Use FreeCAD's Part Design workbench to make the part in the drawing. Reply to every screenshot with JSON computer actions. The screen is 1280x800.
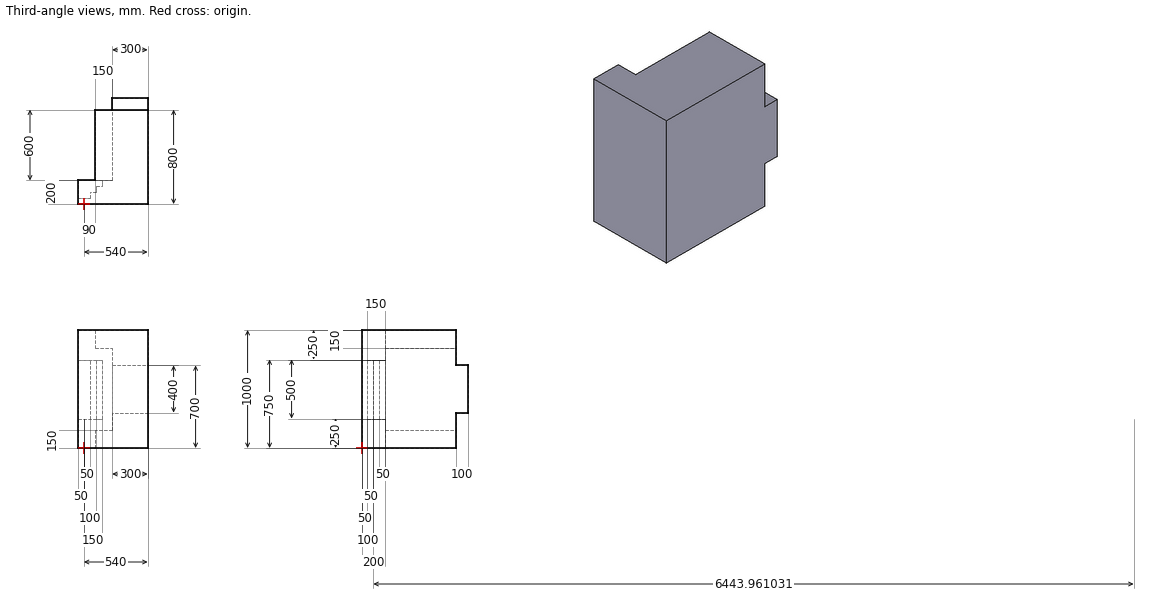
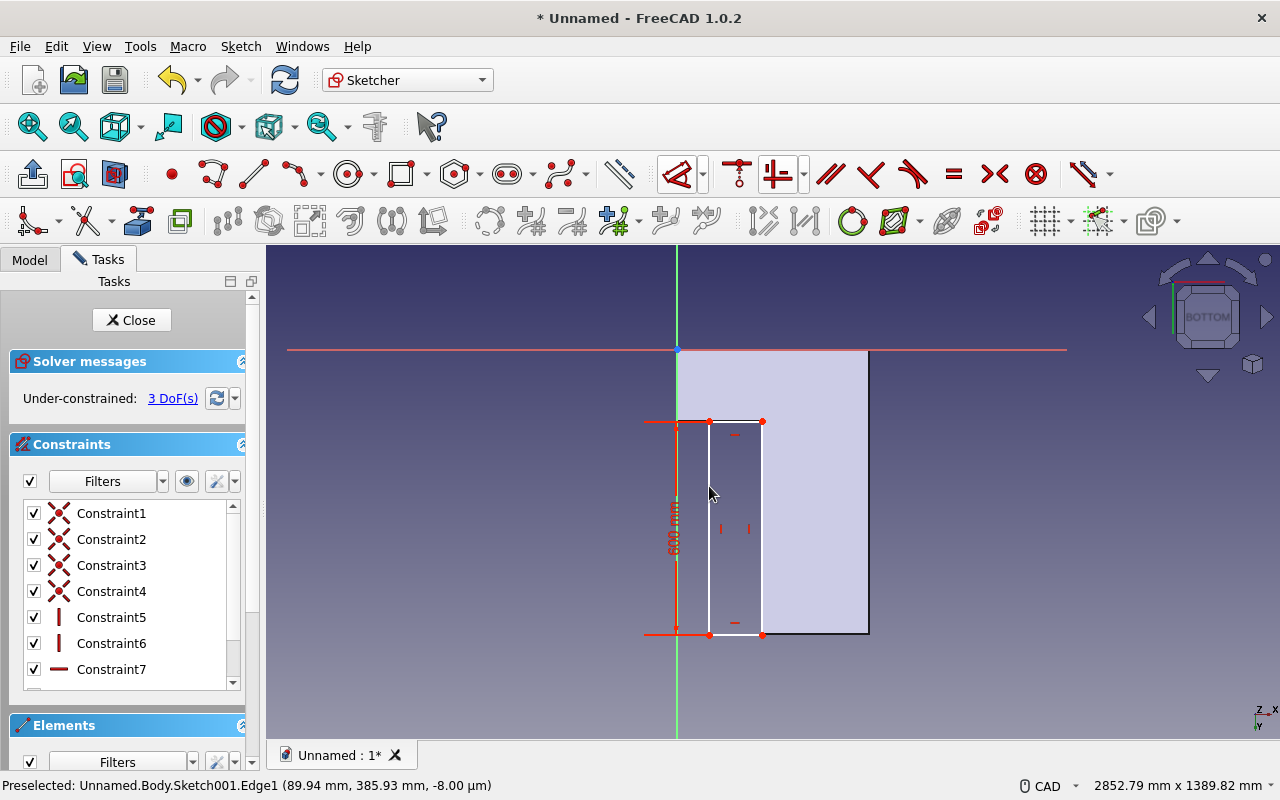
{"action": "left_click", "coordinate": [725, 635]}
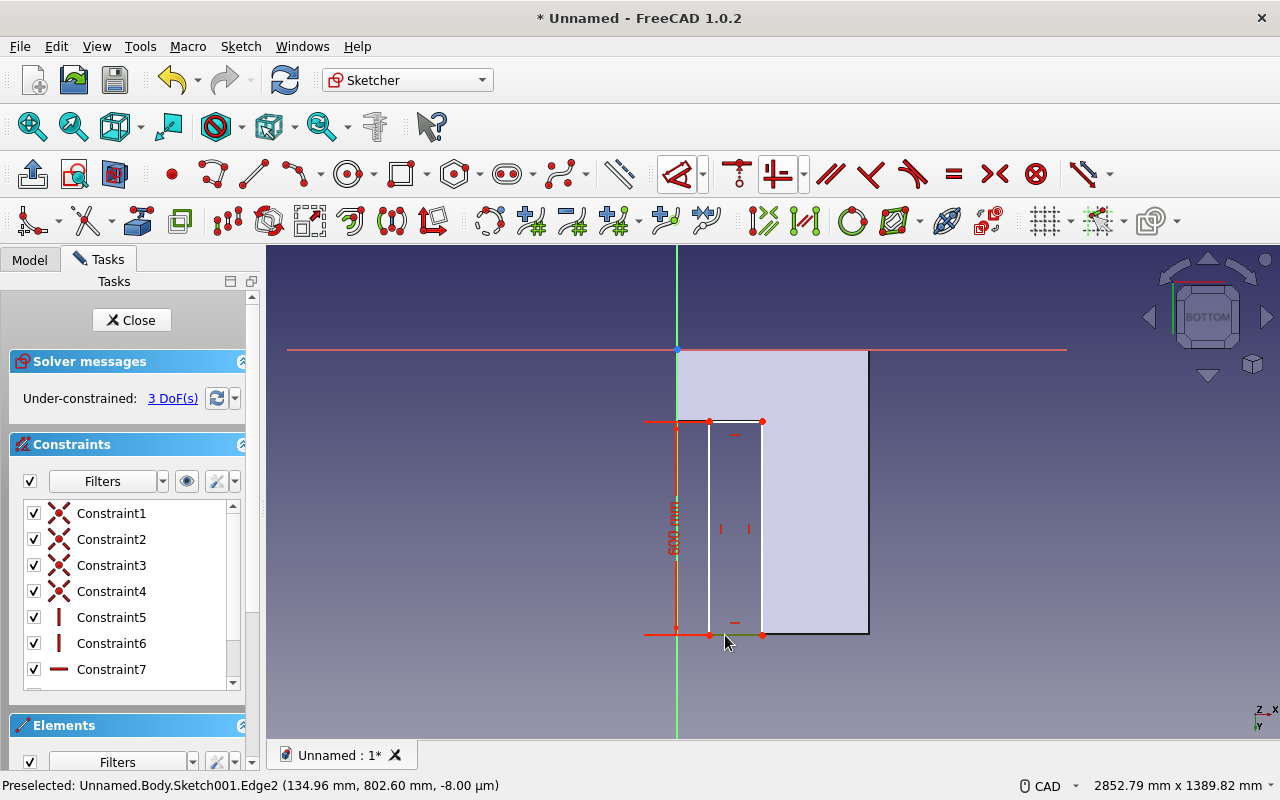
{"action": "left_click", "coordinate": [702, 174]}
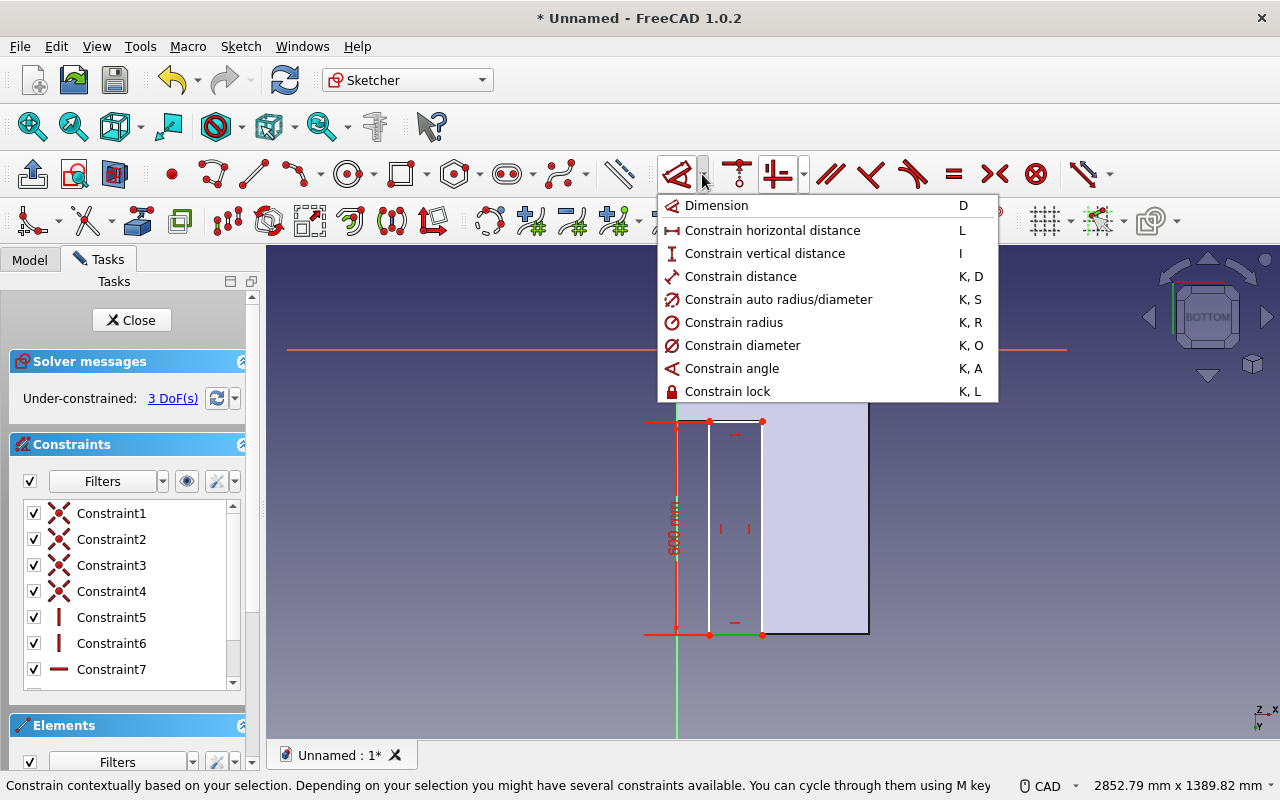
{"action": "left_click", "coordinate": [828, 230]}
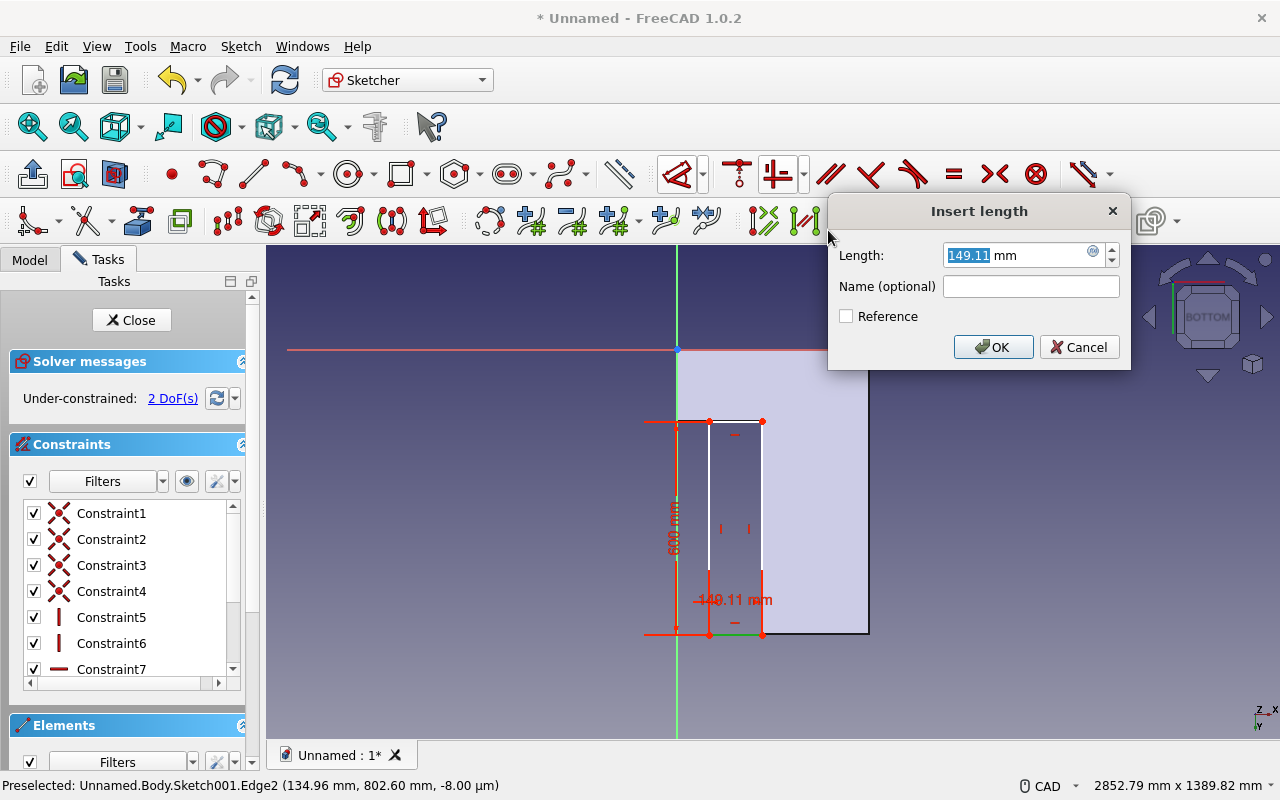
{"action": "type", "text": "150"}
{"action": "key", "text": "Return"}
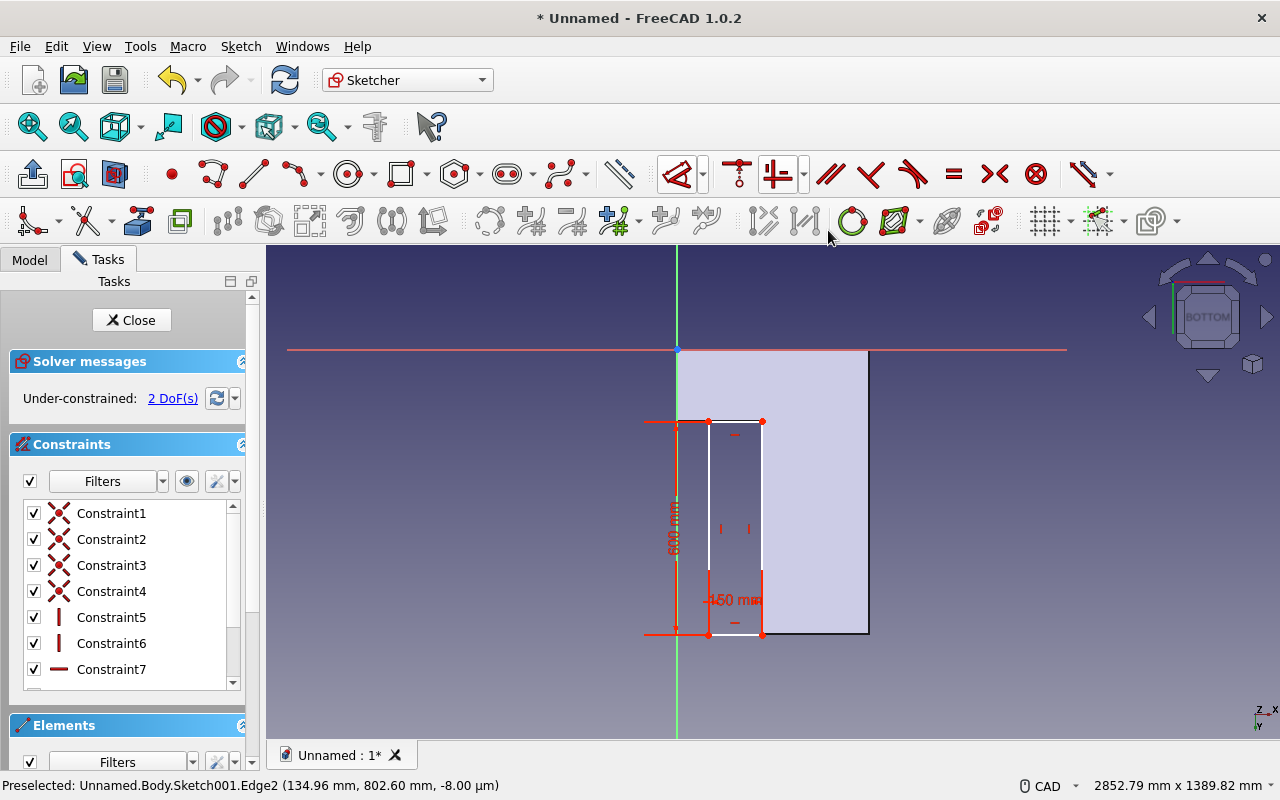
{"action": "scroll", "coordinate": [709, 422], "scroll_direction": "up", "scroll_amount": 2}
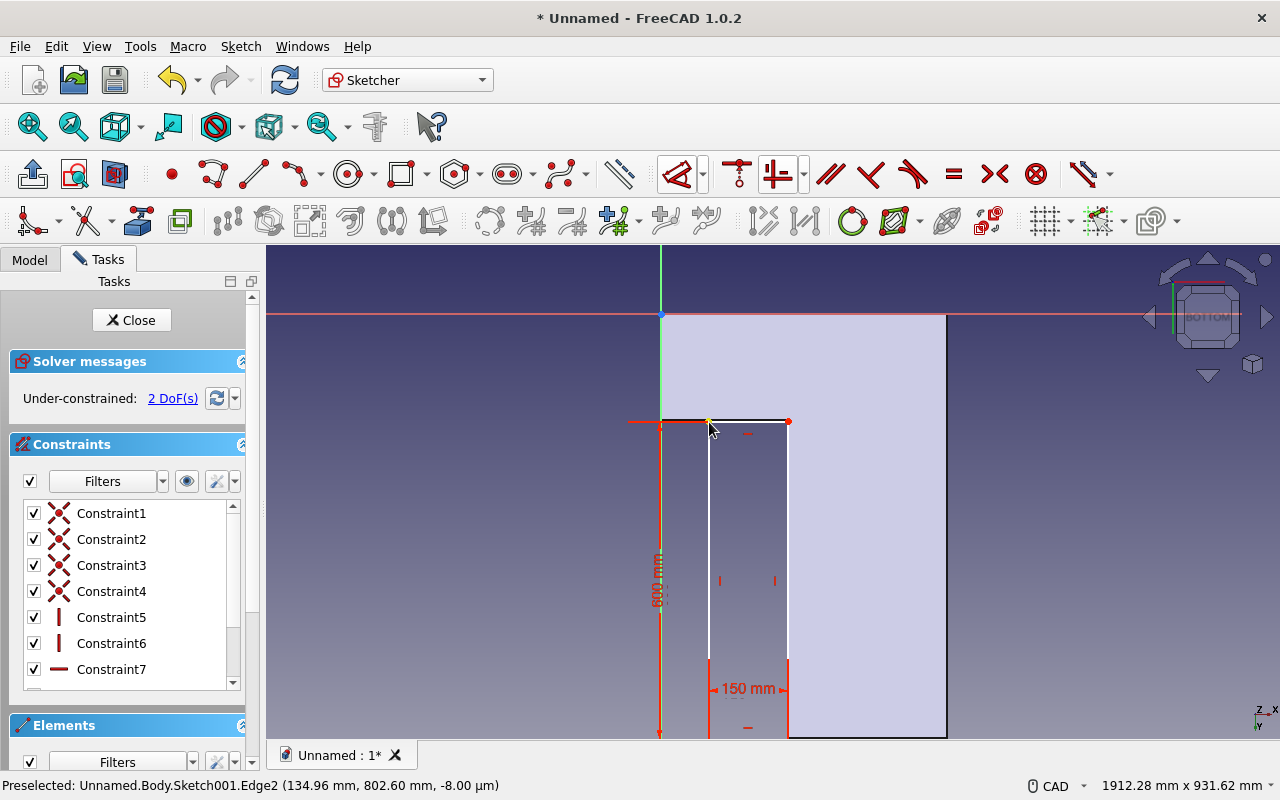
{"action": "left_click", "coordinate": [709, 422]}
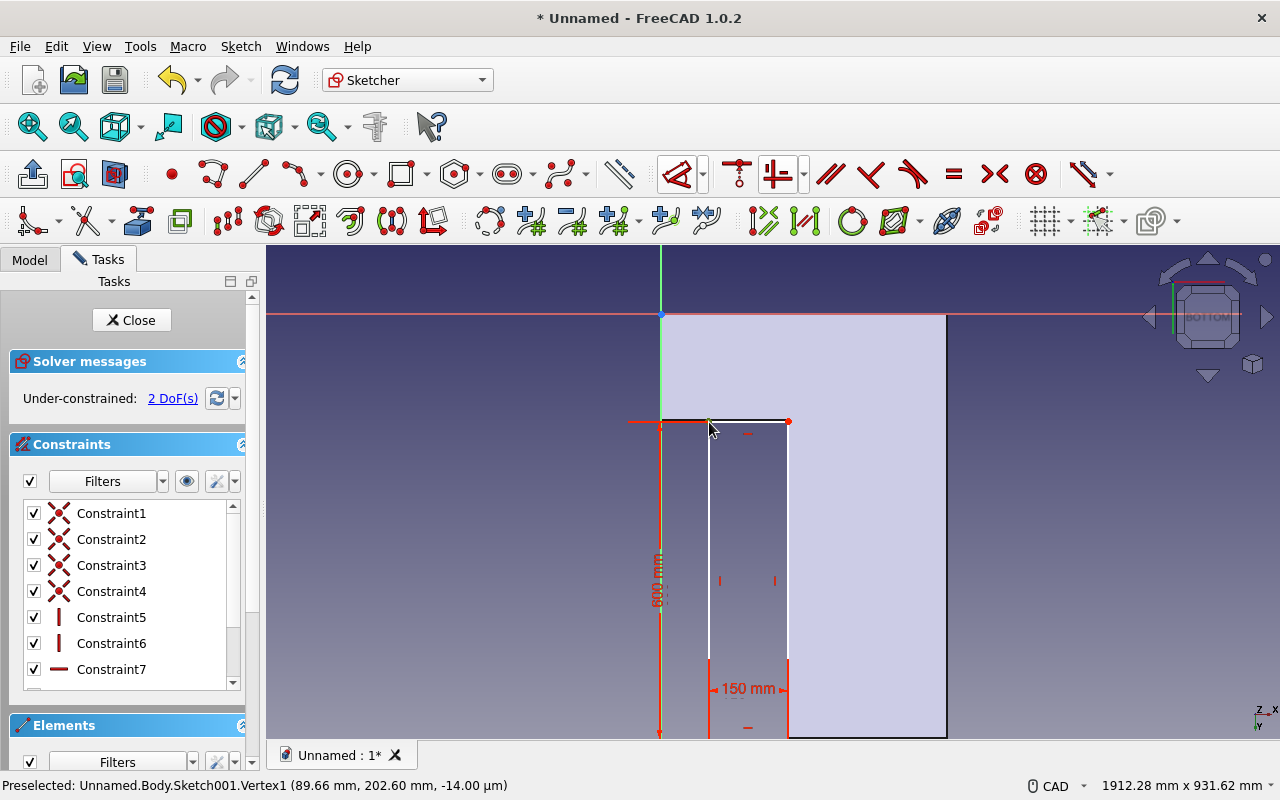
{"action": "key", "text": "l"}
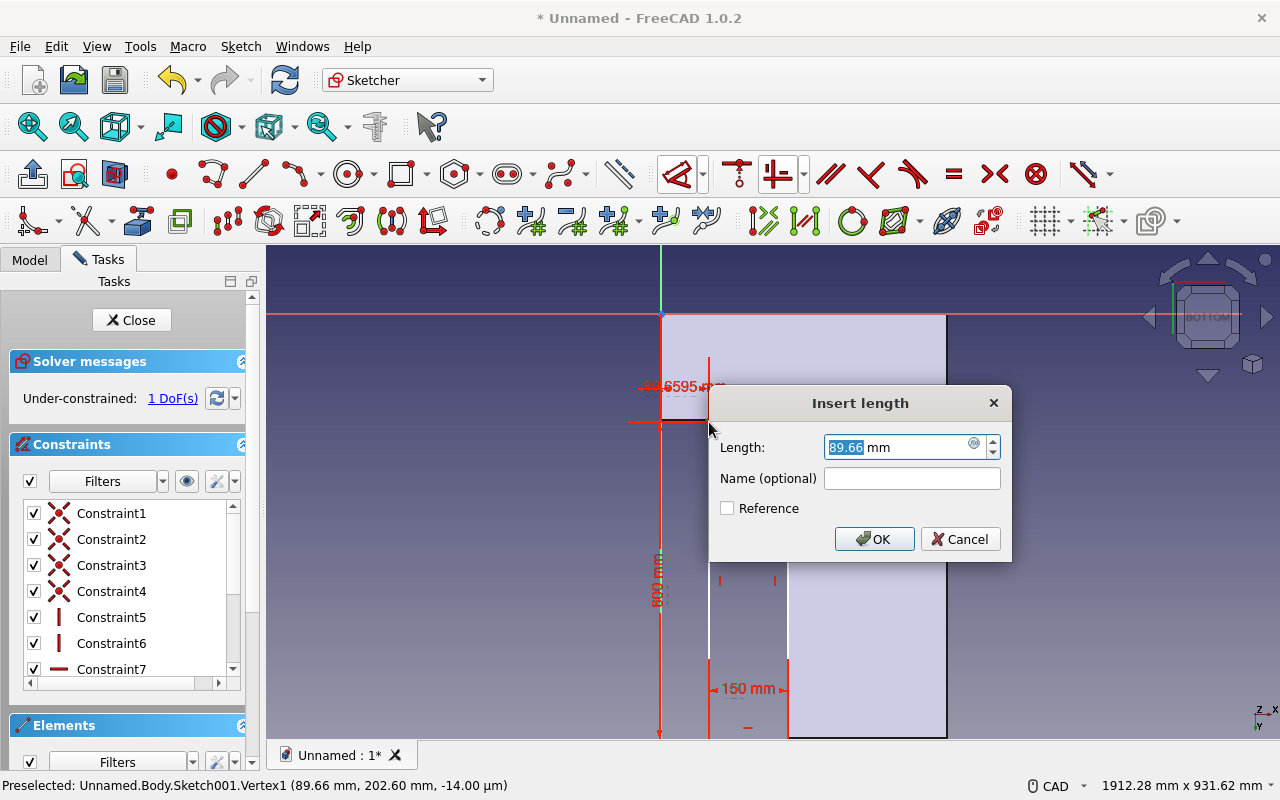
{"action": "type", "text": "90"}
{"action": "key", "text": "Return"}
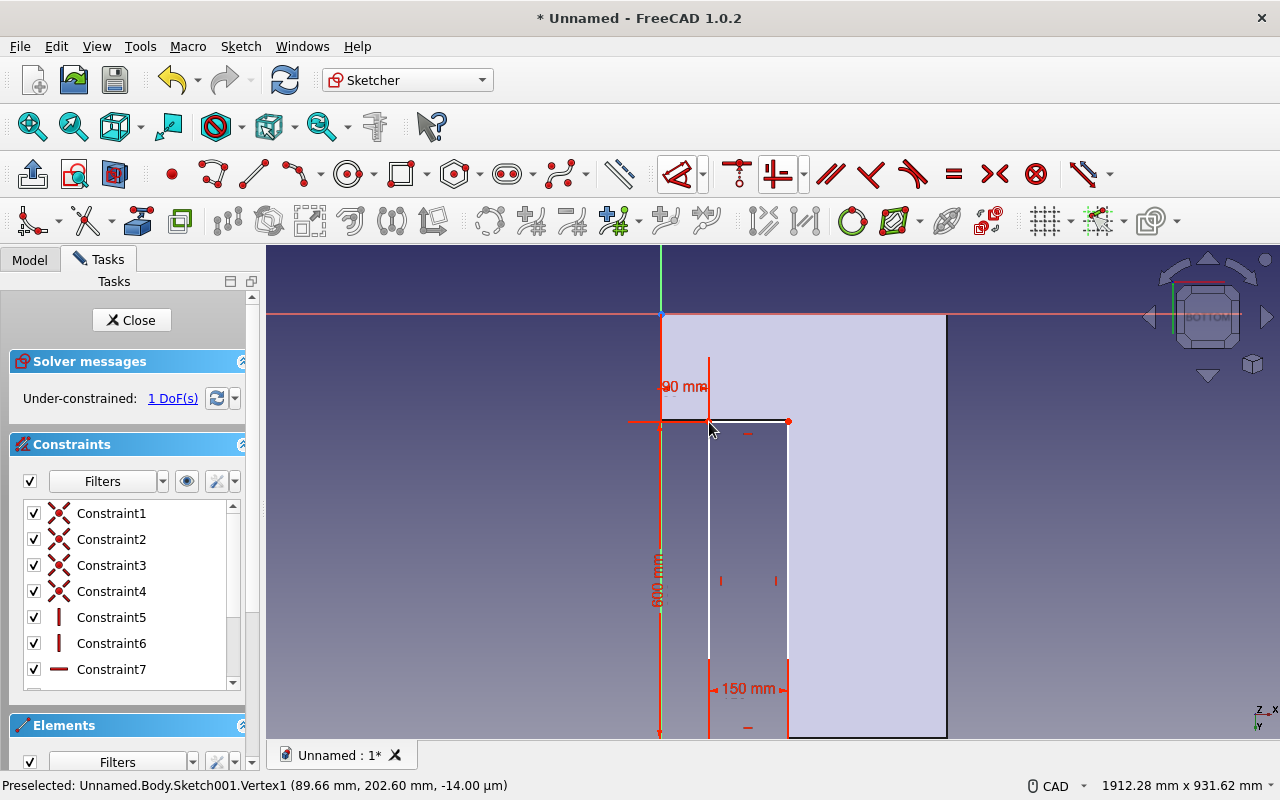
{"action": "left_click", "coordinate": [709, 422]}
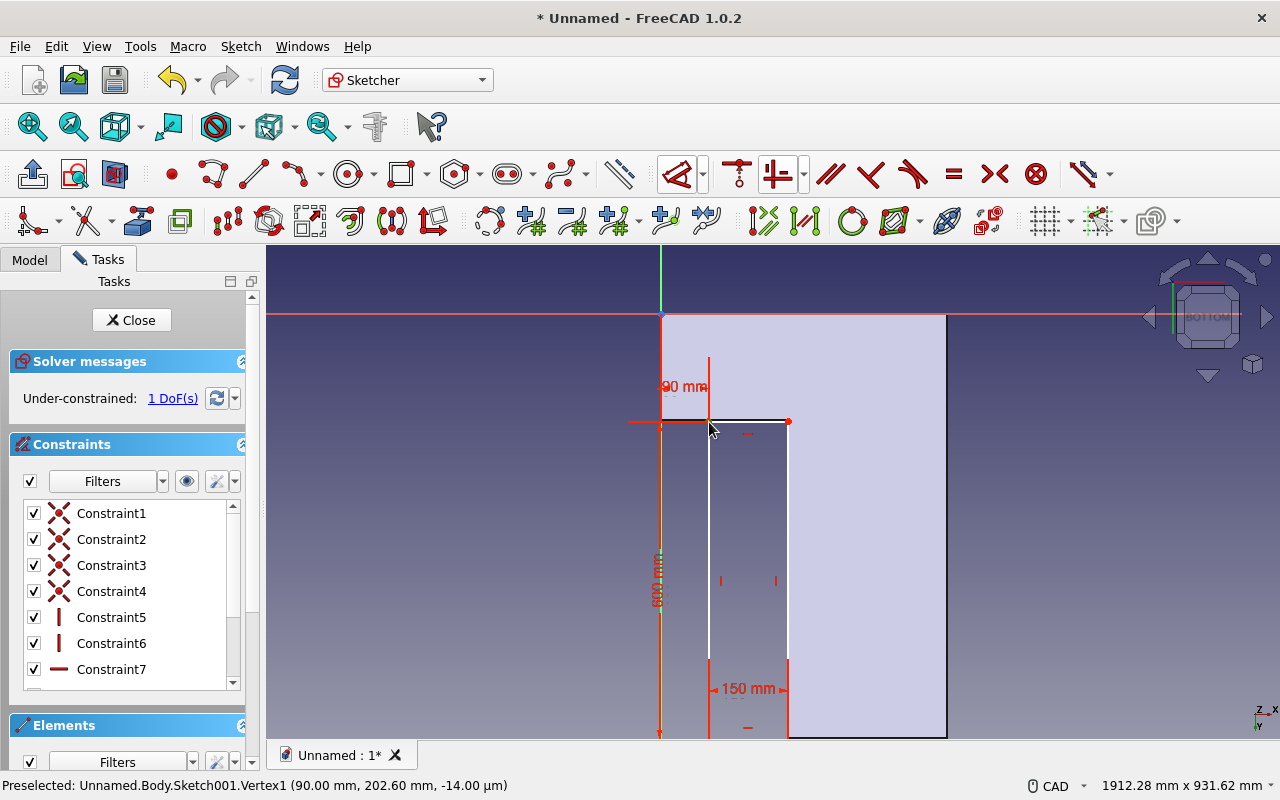
{"action": "key", "text": "i"}